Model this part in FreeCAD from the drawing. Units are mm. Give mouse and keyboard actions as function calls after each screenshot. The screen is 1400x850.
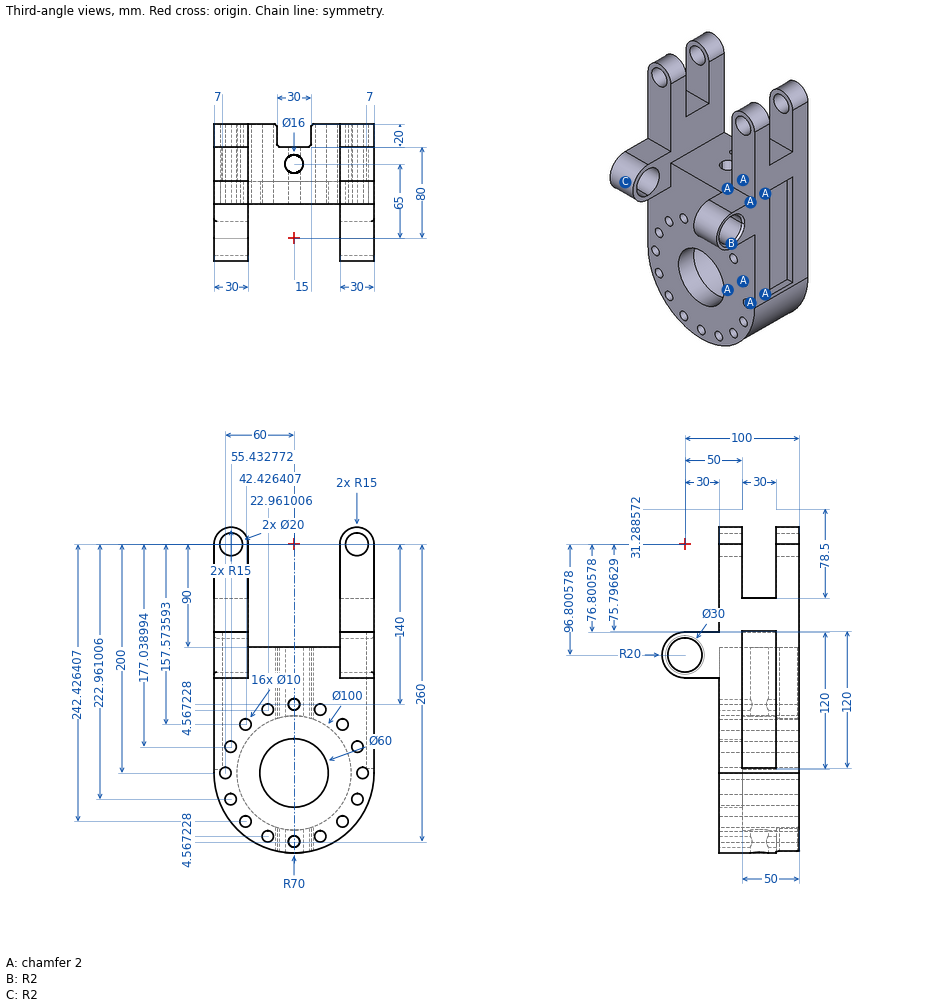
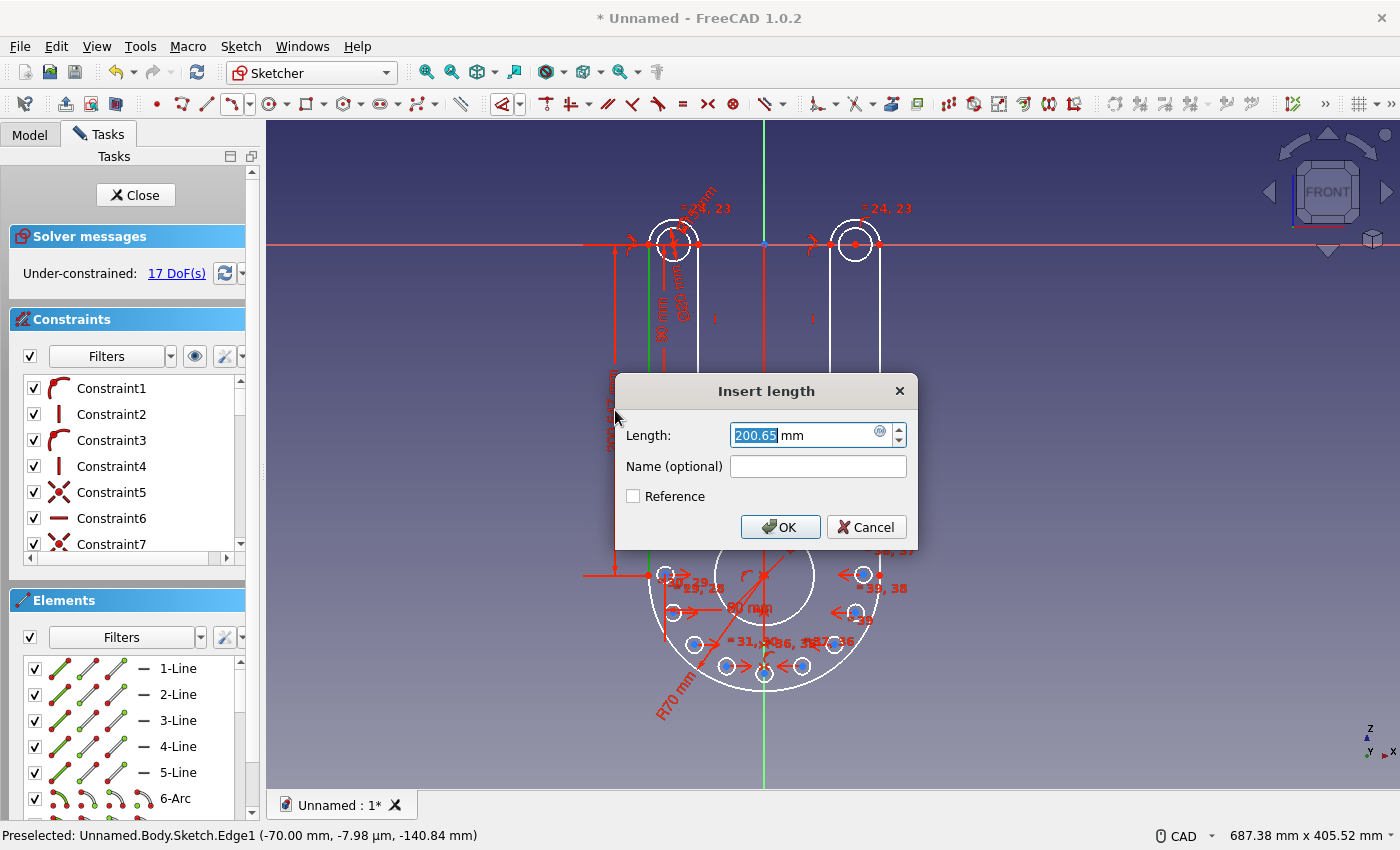
text(200)
key(Return)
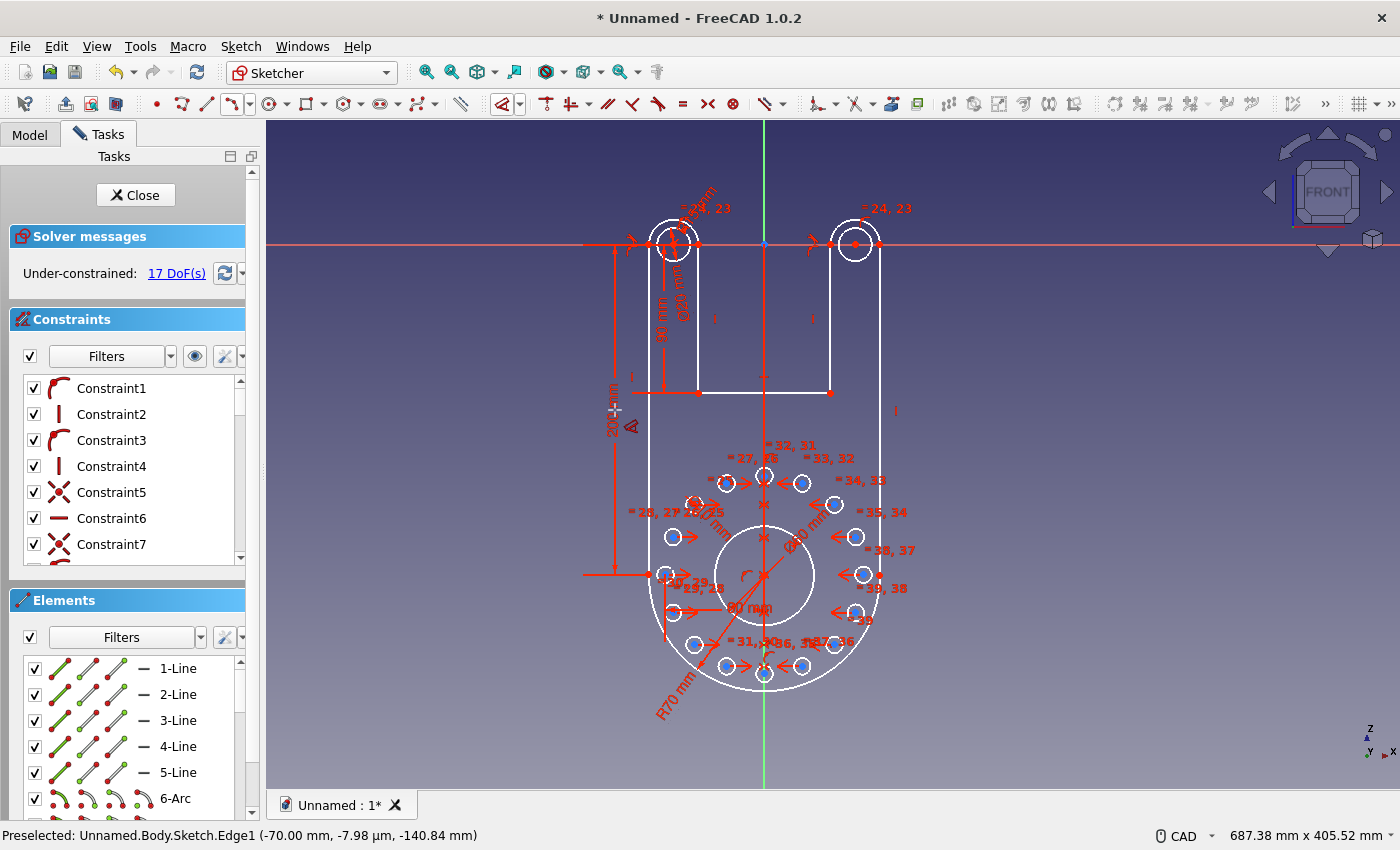
click(880, 344)
click(914, 410)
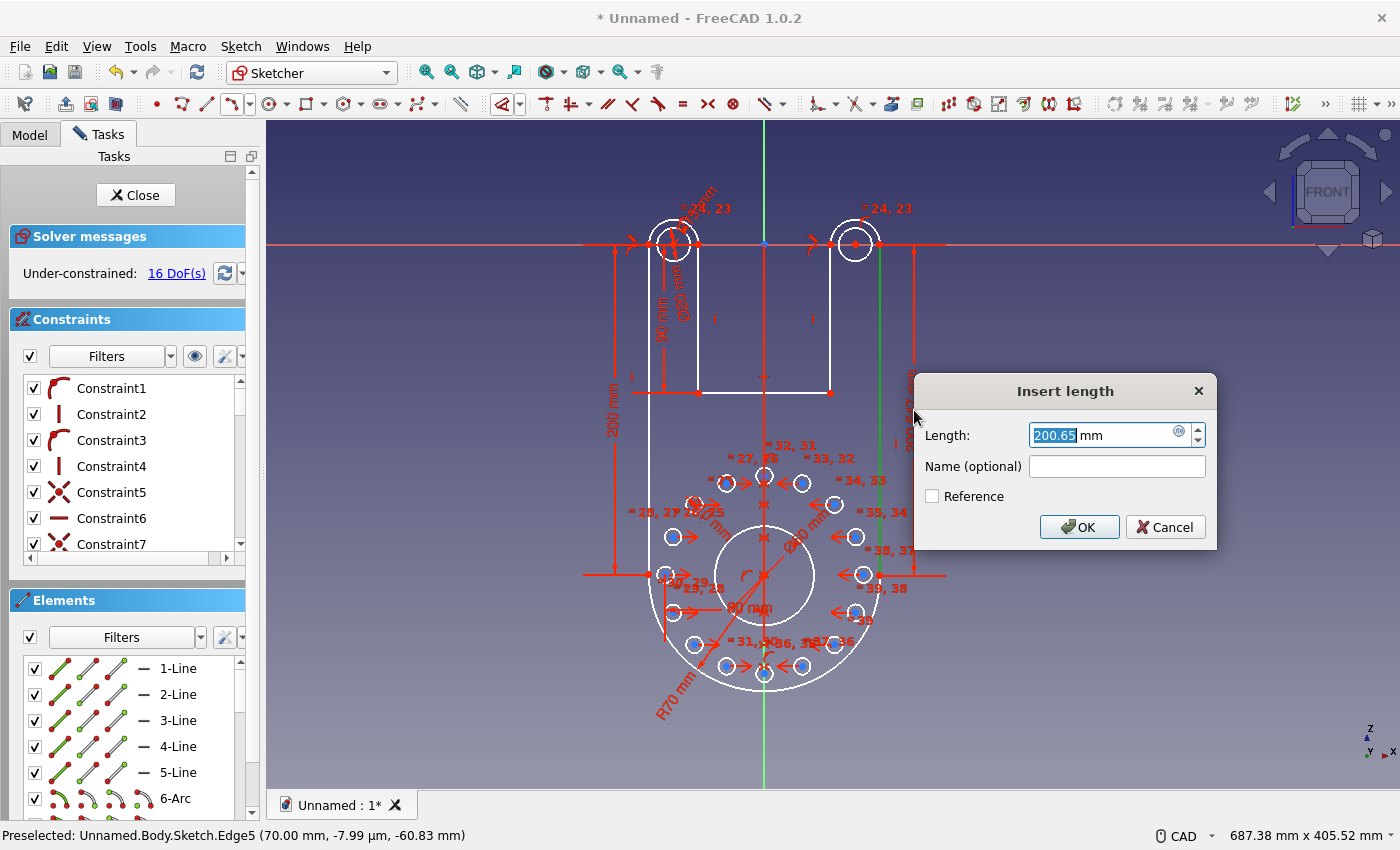
text(200)
key(Return)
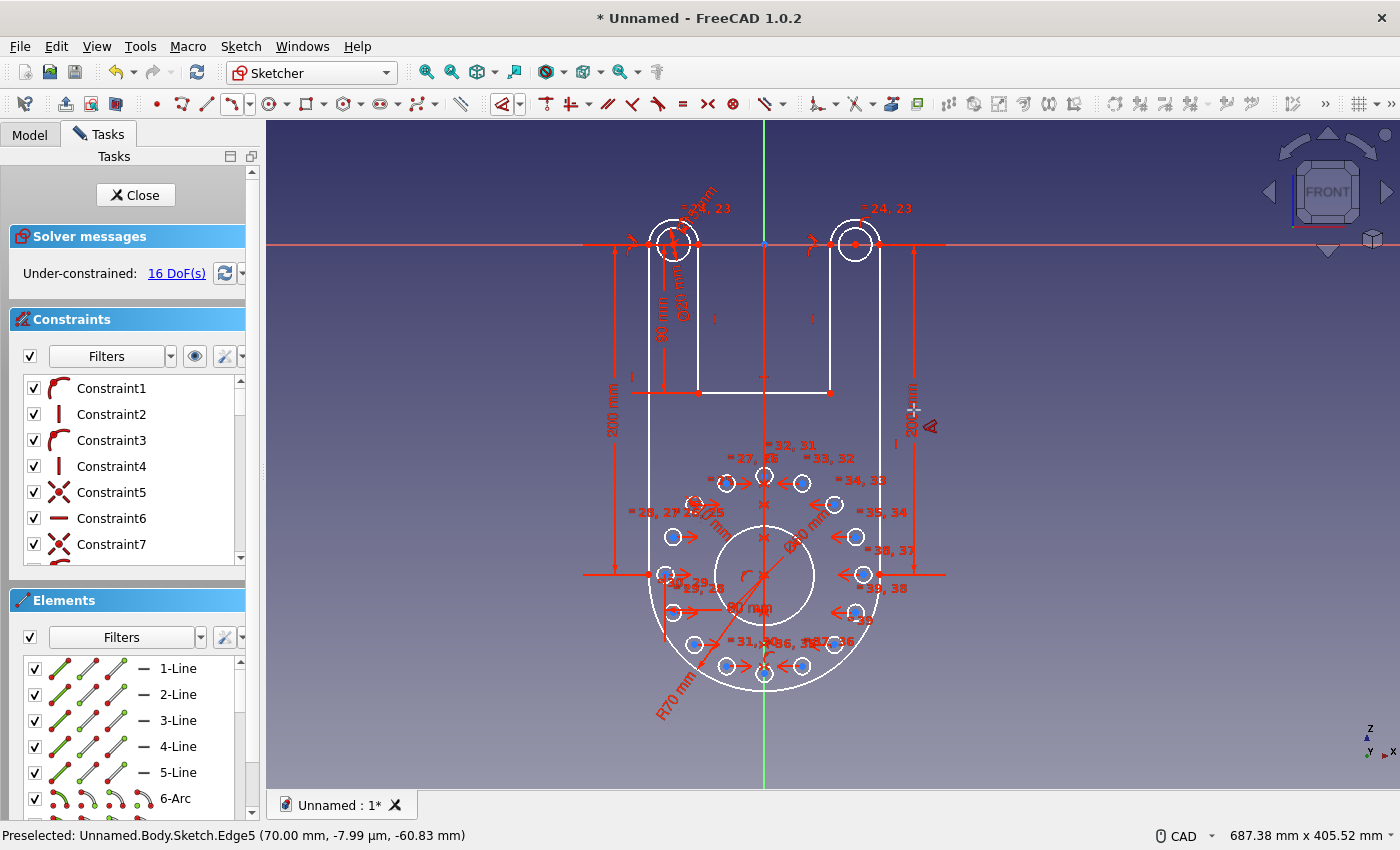
click(665, 575)
click(631, 486)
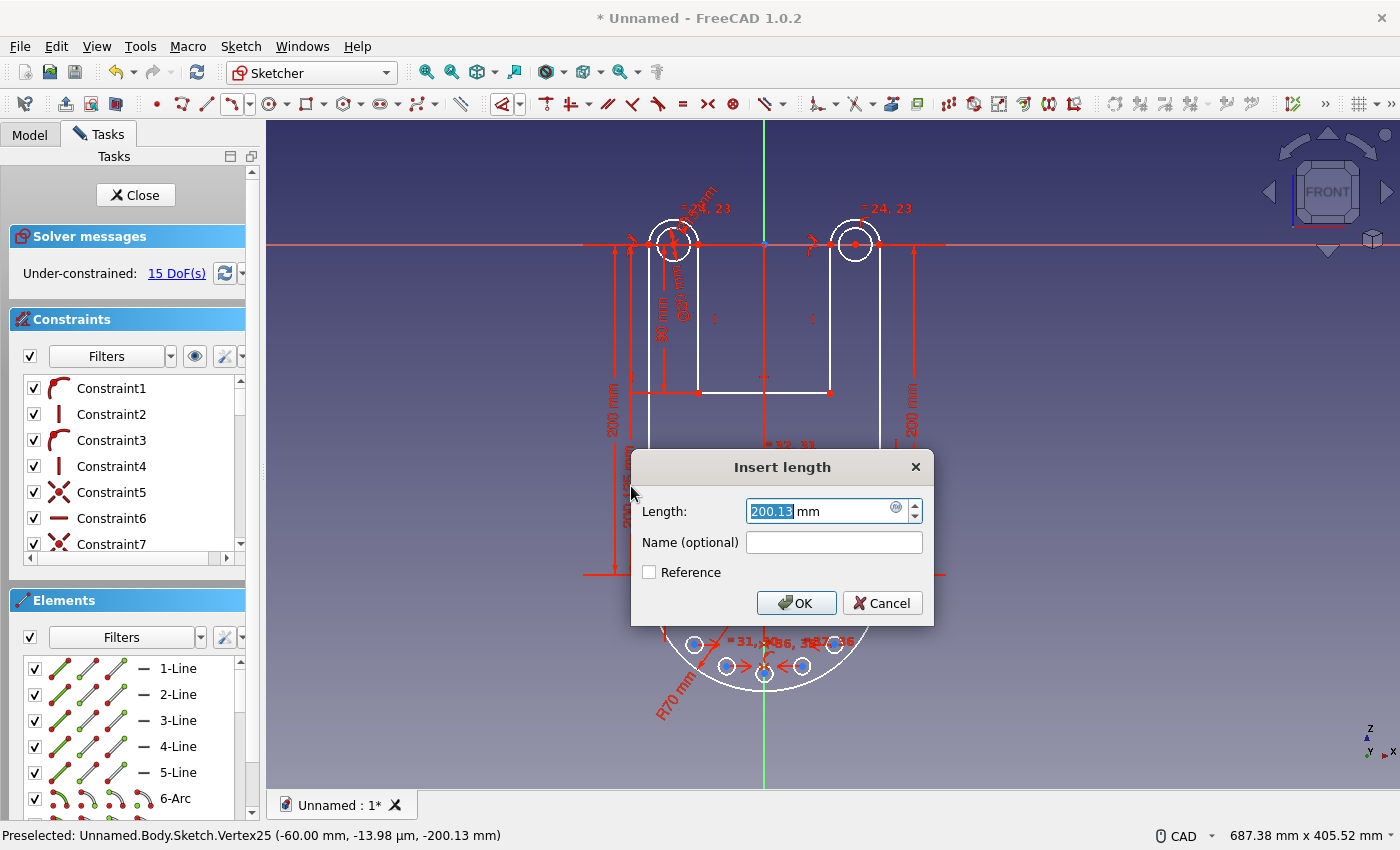
text(200)
key(Return)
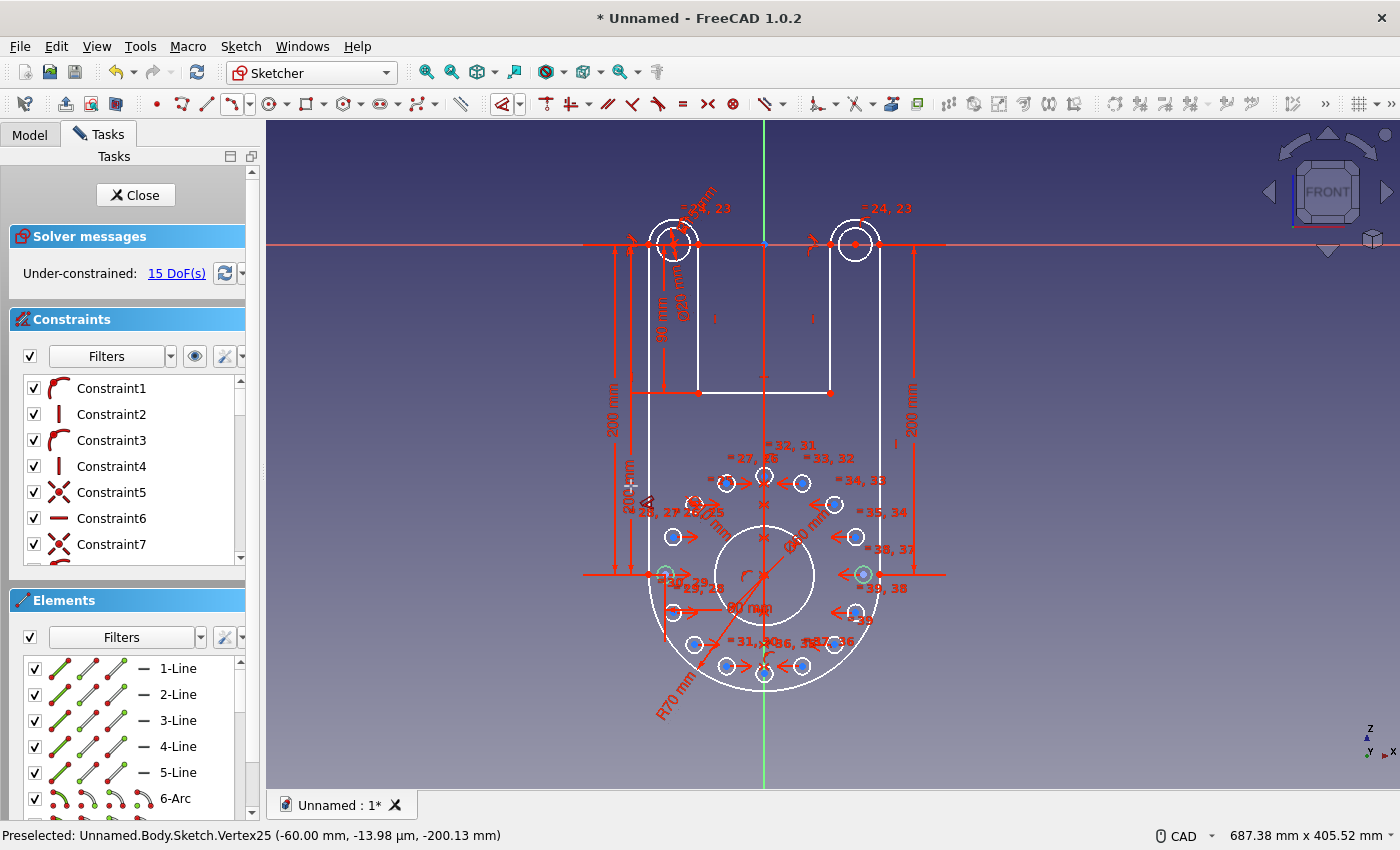
click(764, 476)
click(798, 360)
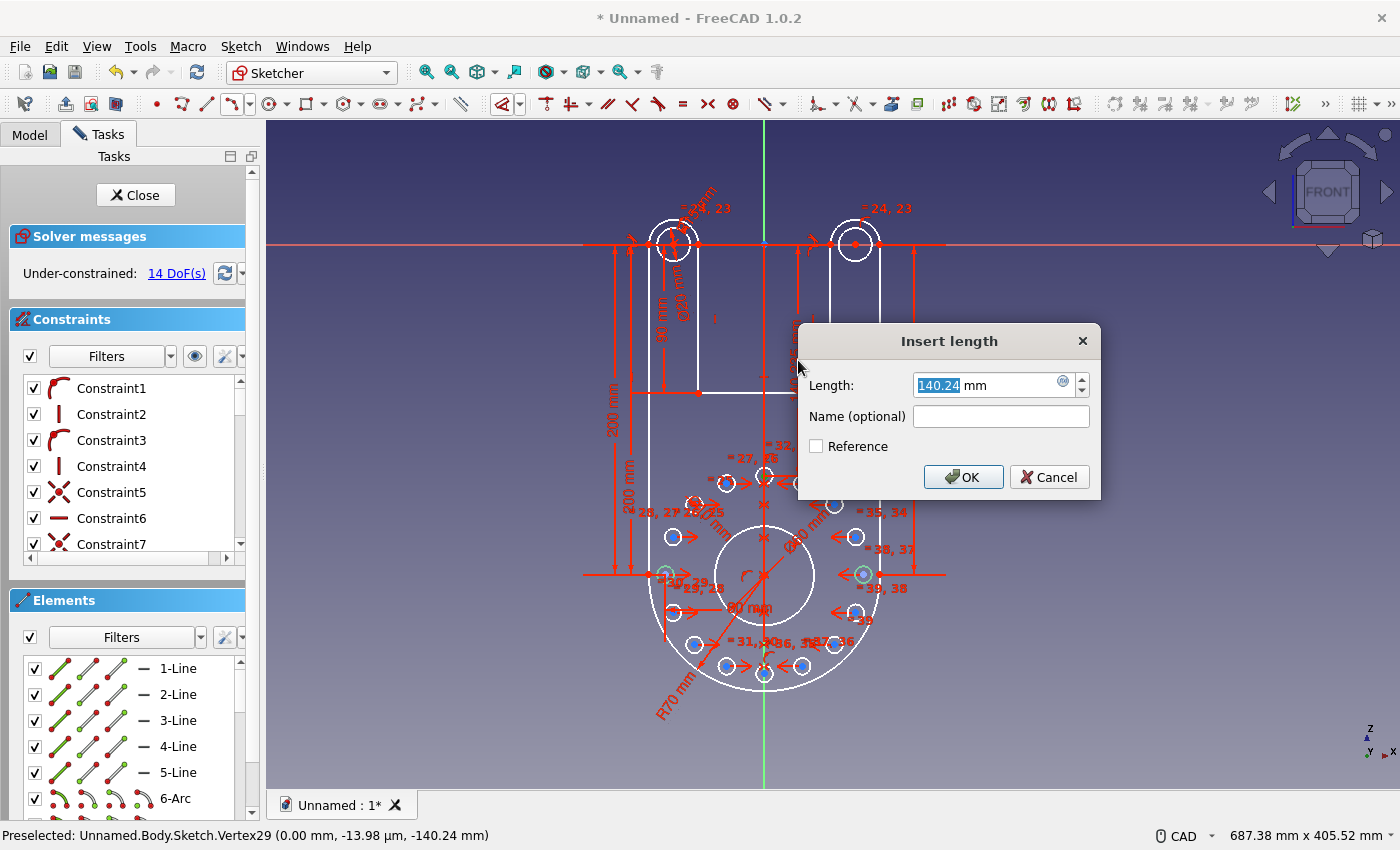
text(140)
key(Return)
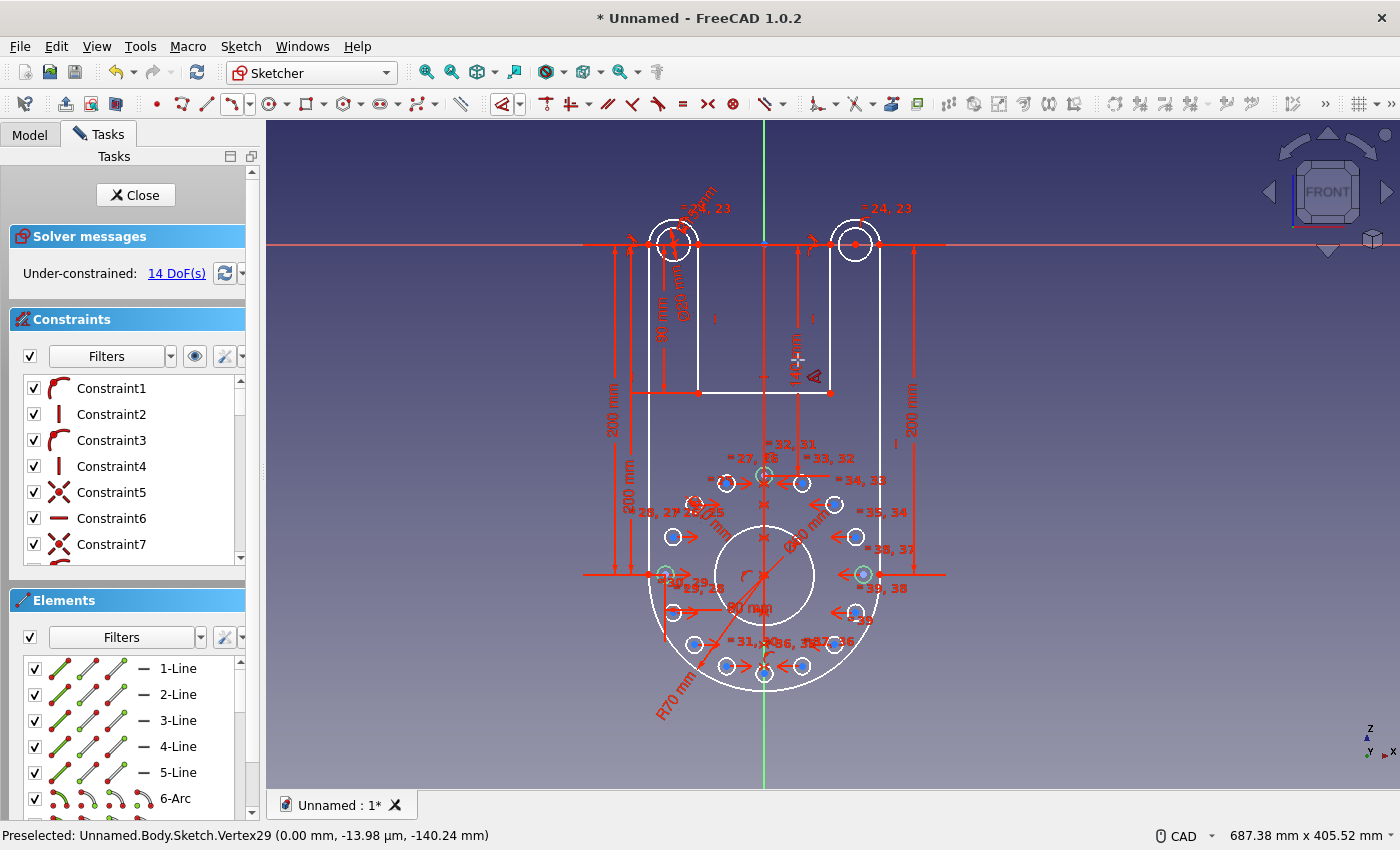
click(764, 576)
click(798, 410)